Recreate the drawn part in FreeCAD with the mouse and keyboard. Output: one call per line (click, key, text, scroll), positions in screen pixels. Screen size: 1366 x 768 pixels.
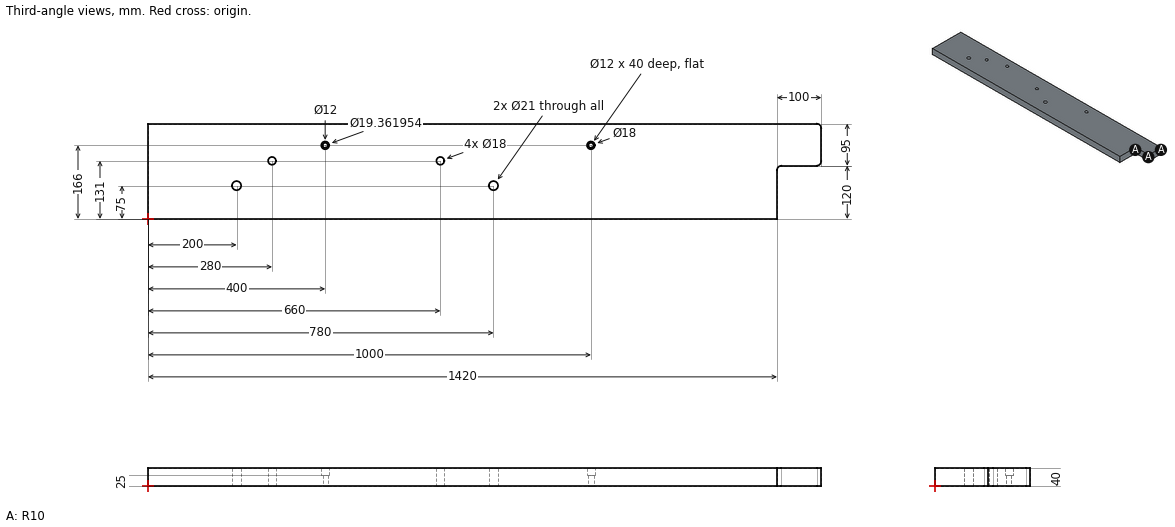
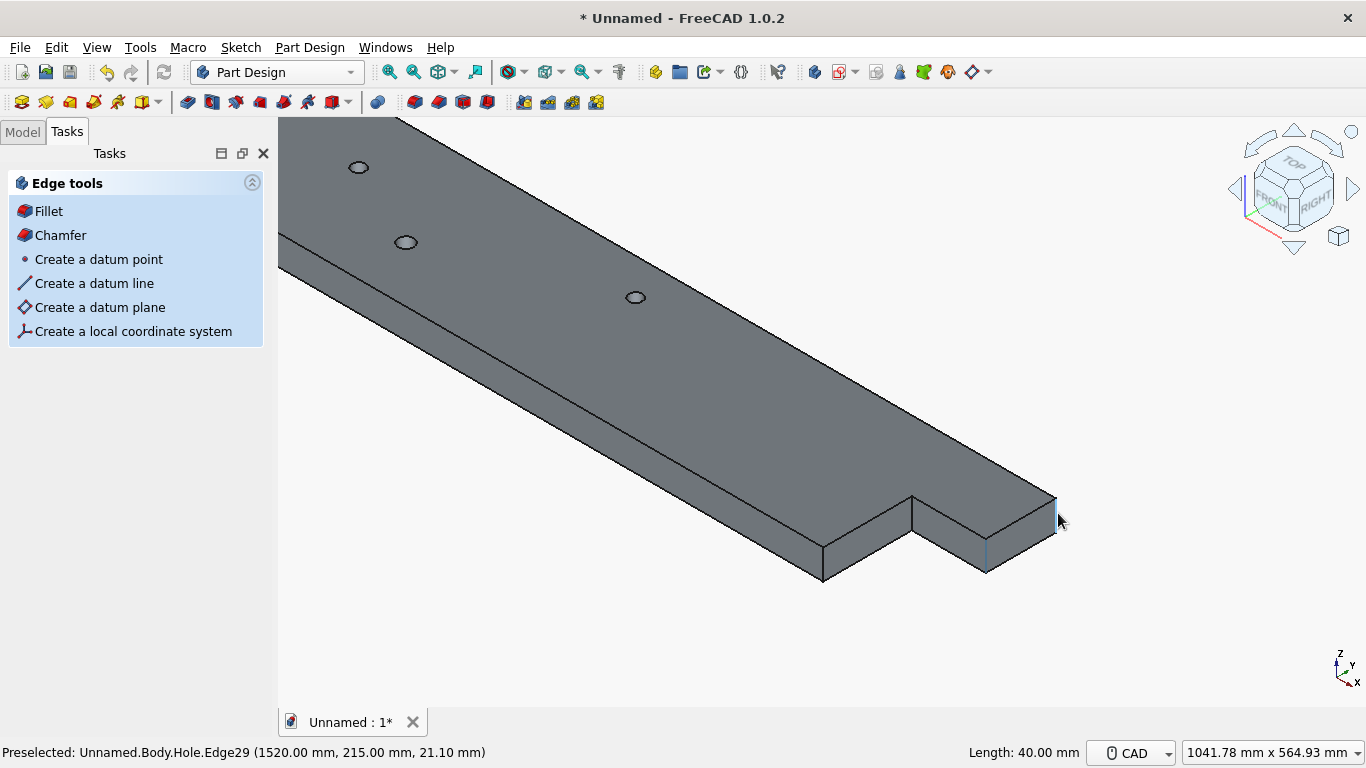
key(v)
key(f)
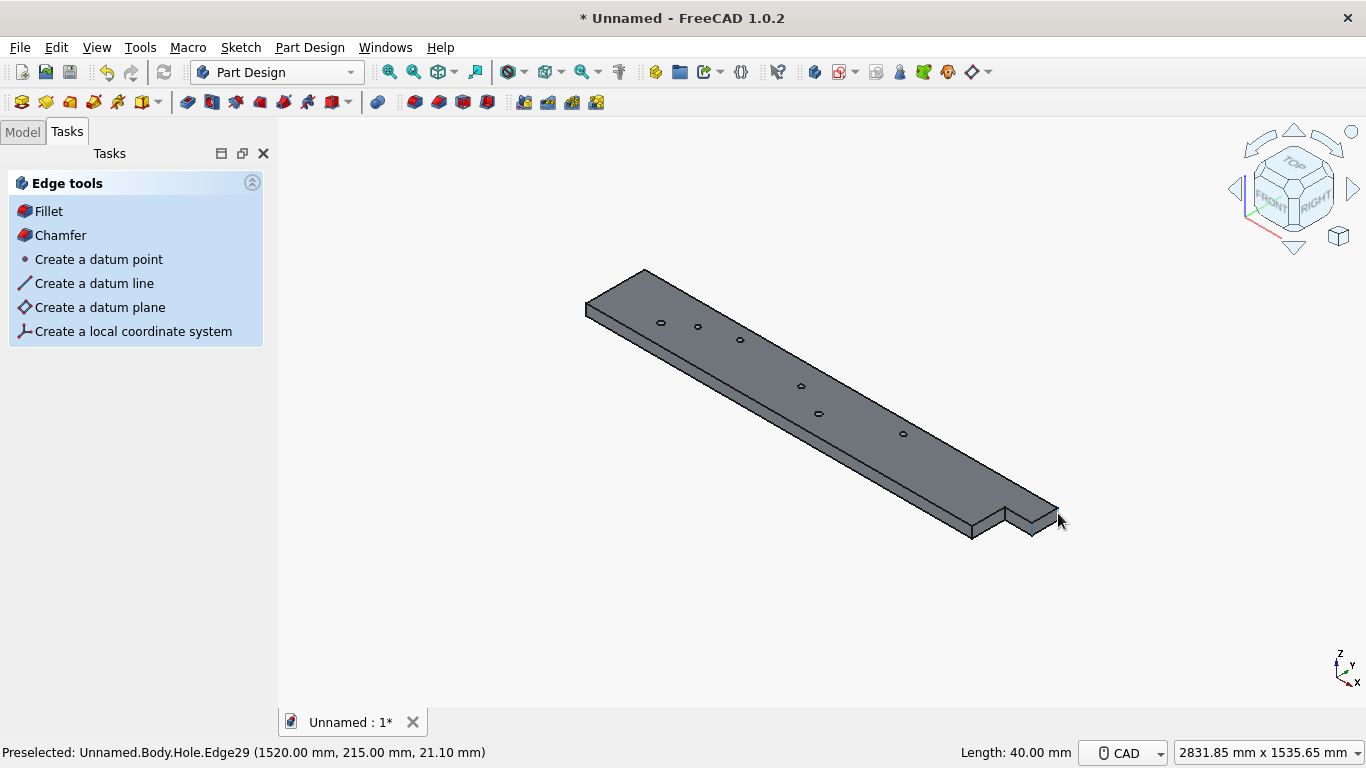
key(2)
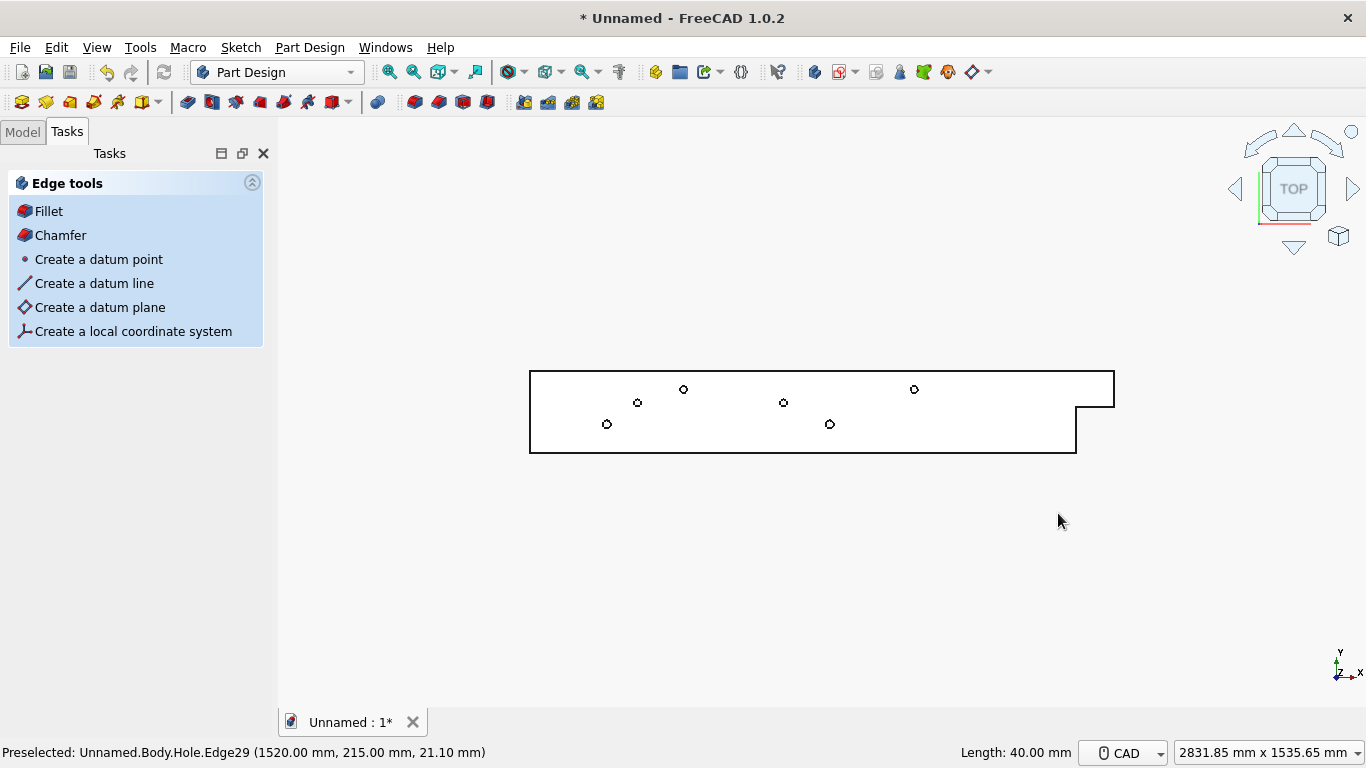
scroll(1114, 370, up, 5)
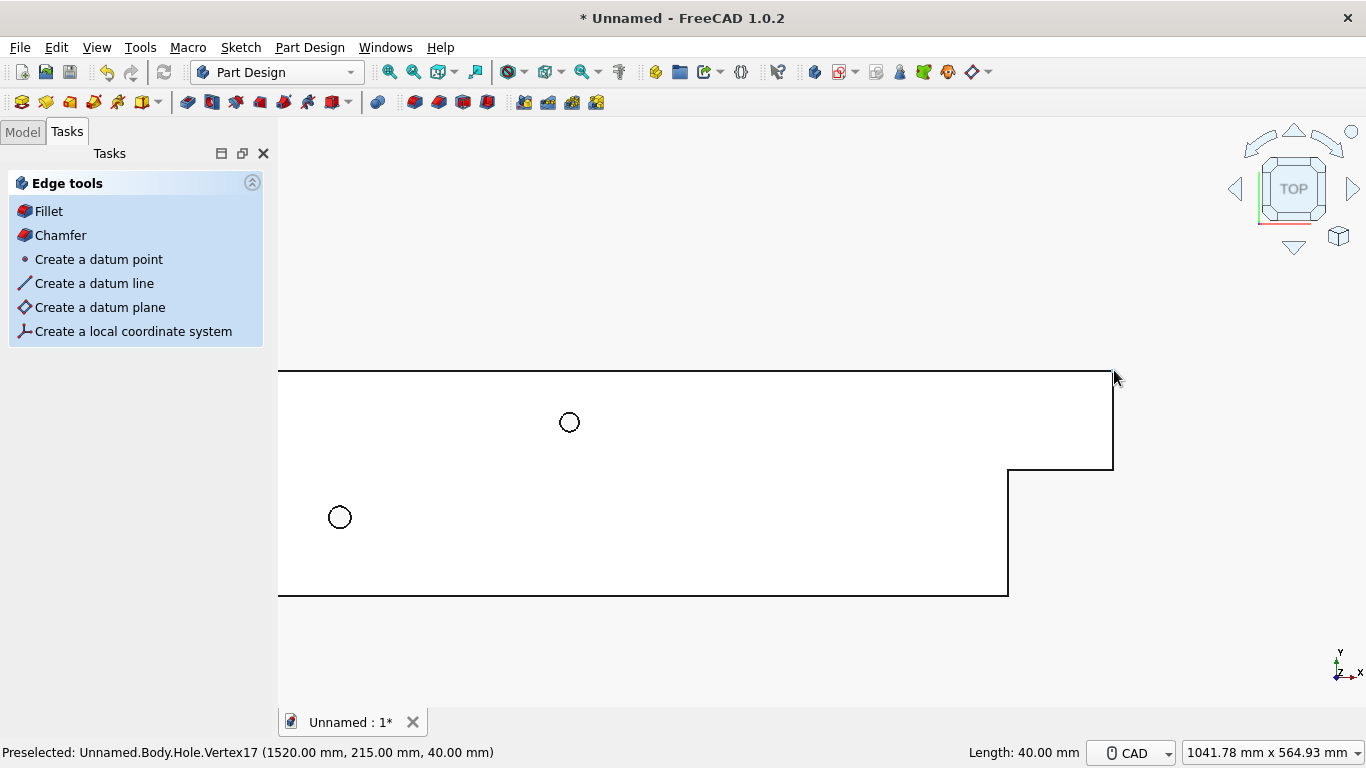
key(v)
key(f)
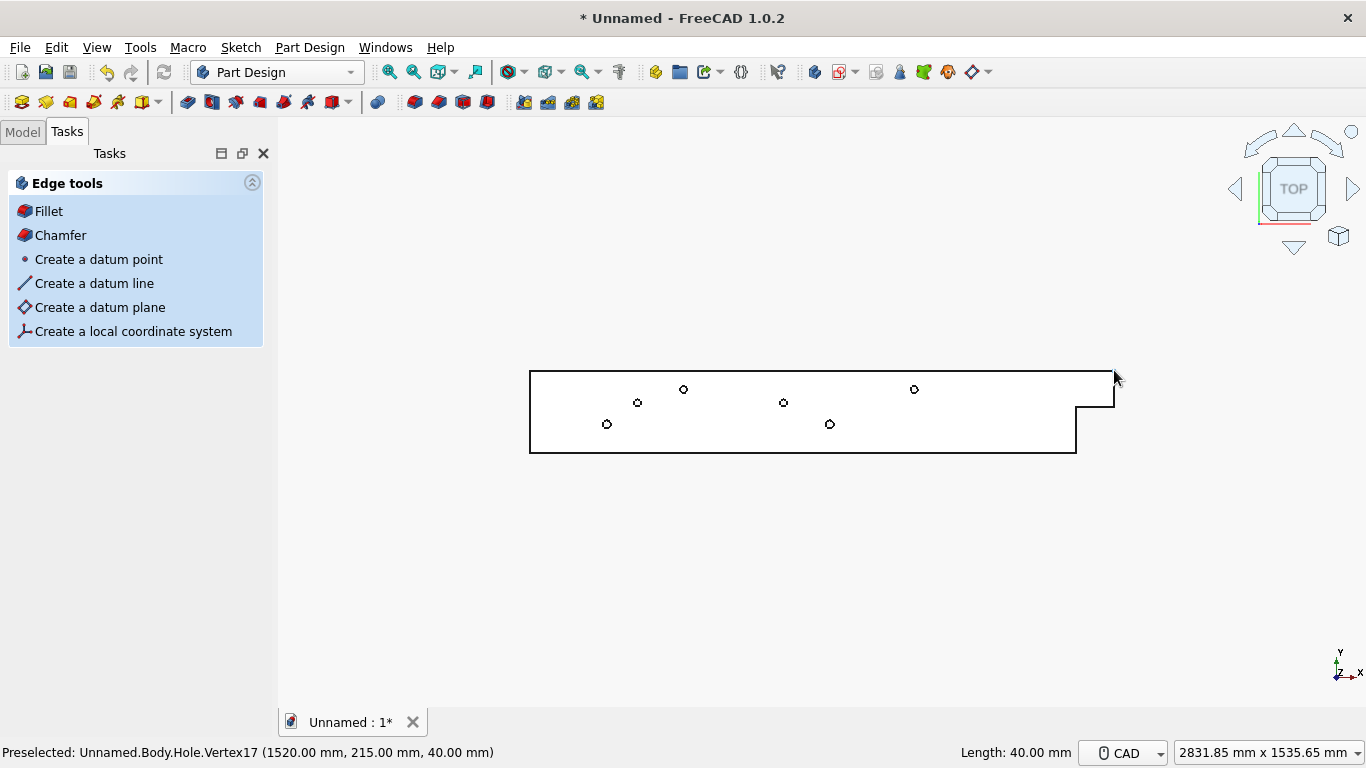
key(1)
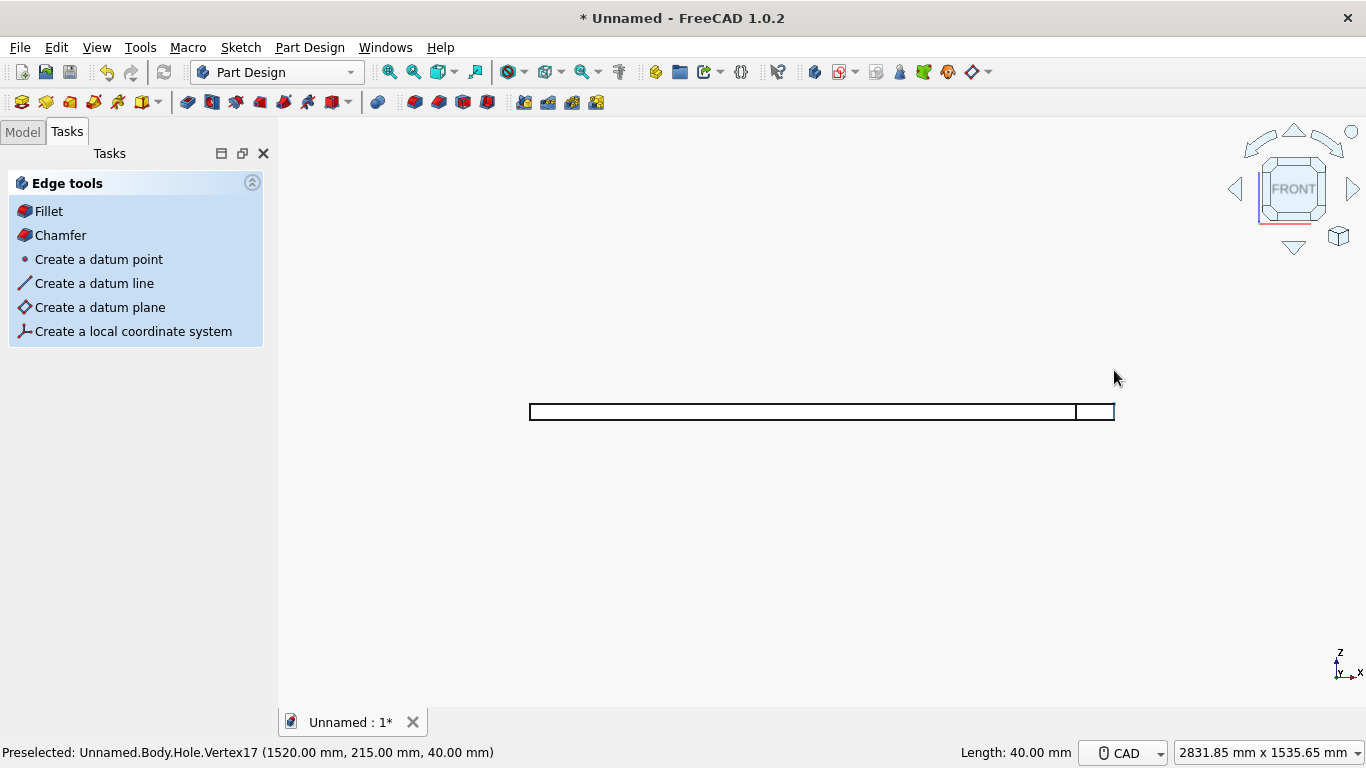
scroll(1114, 411, up, 5)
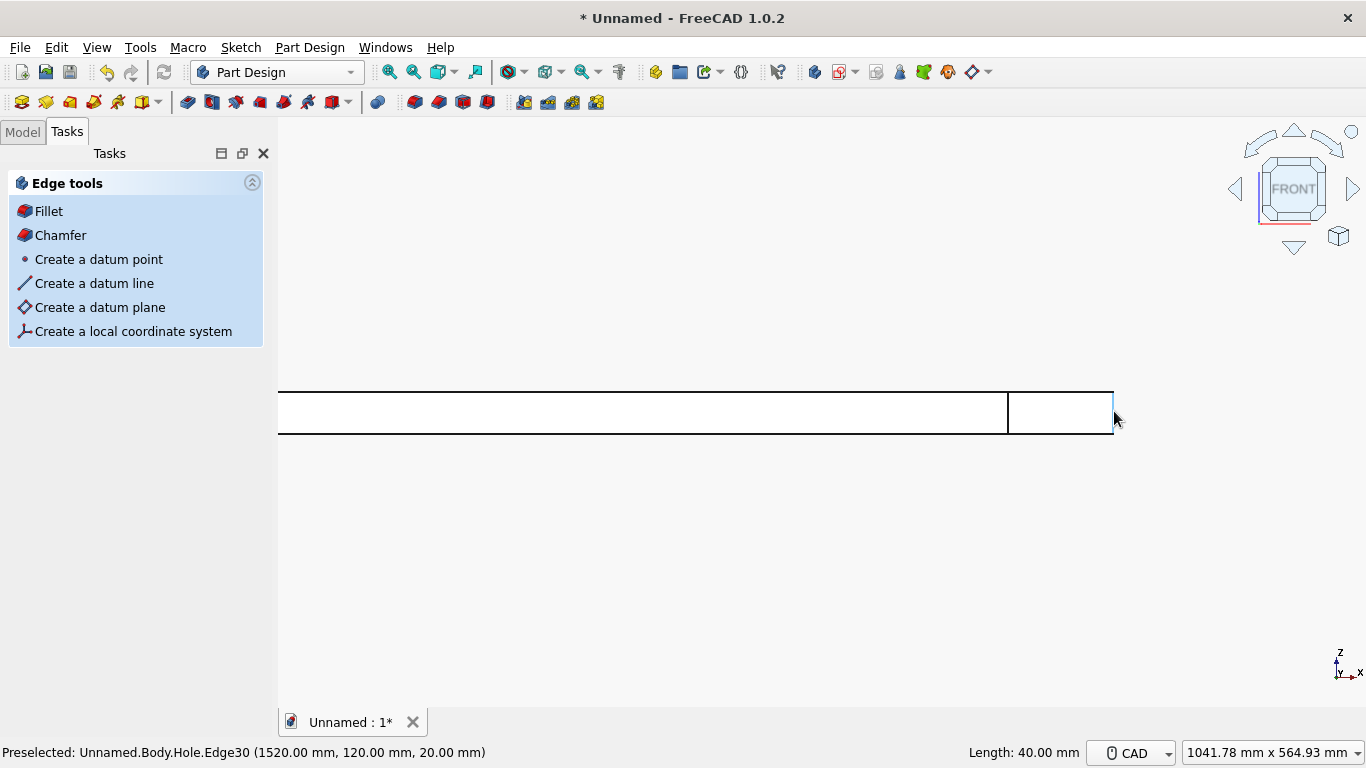
key(v)
key(f)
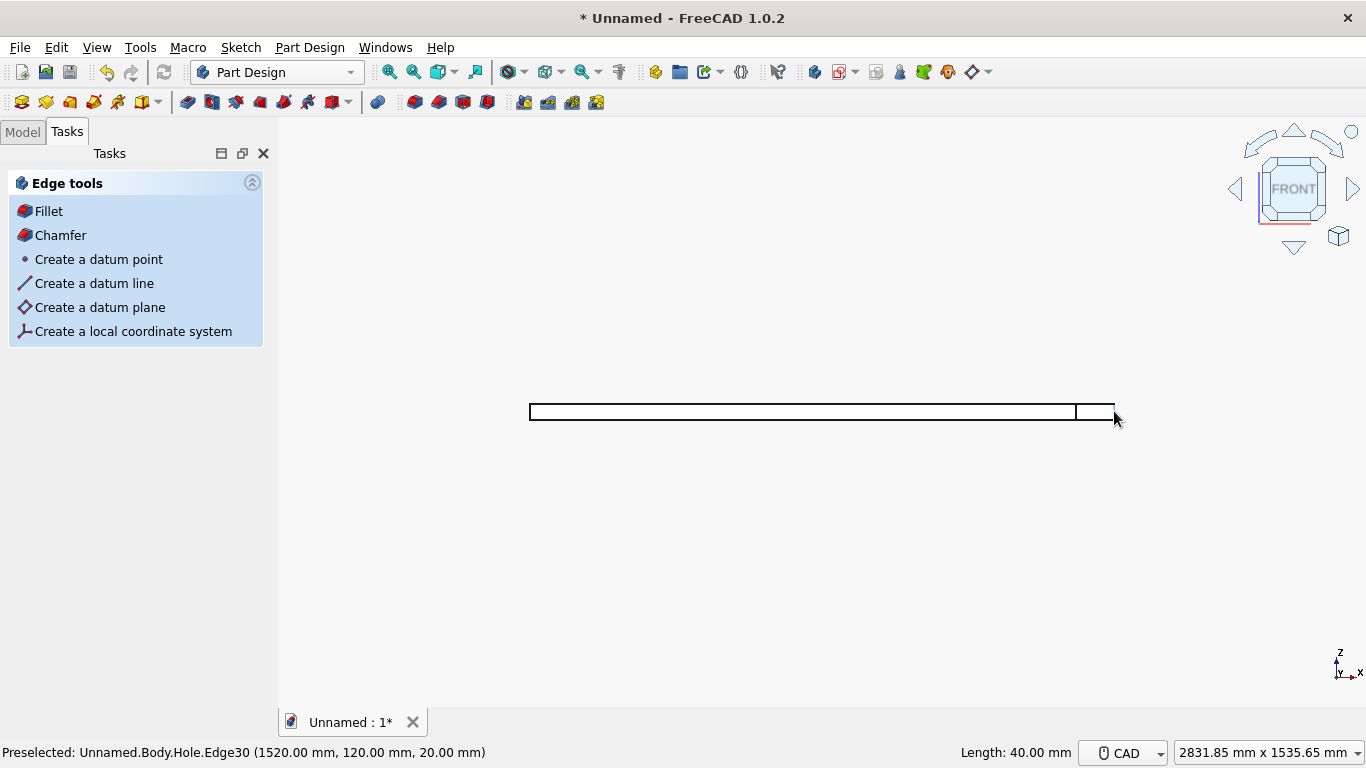
key(3)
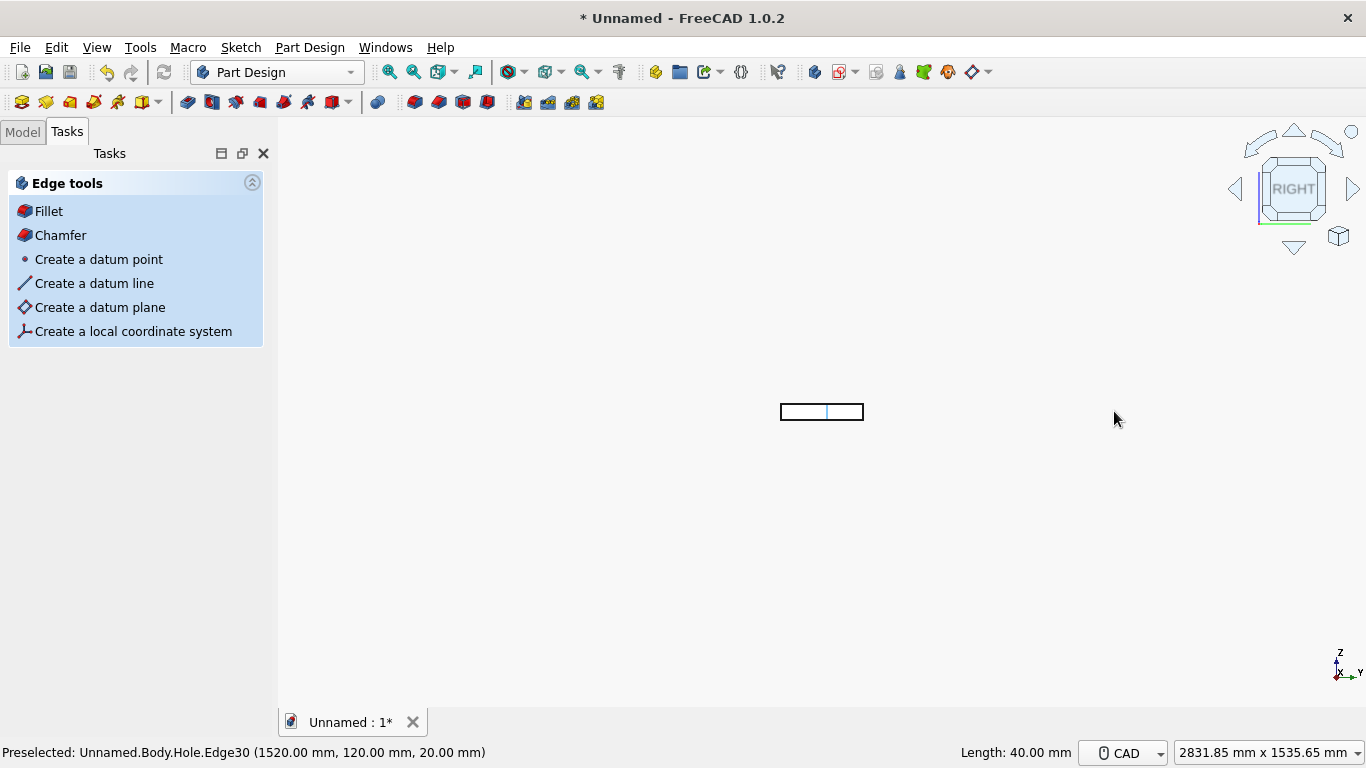
click(390, 72)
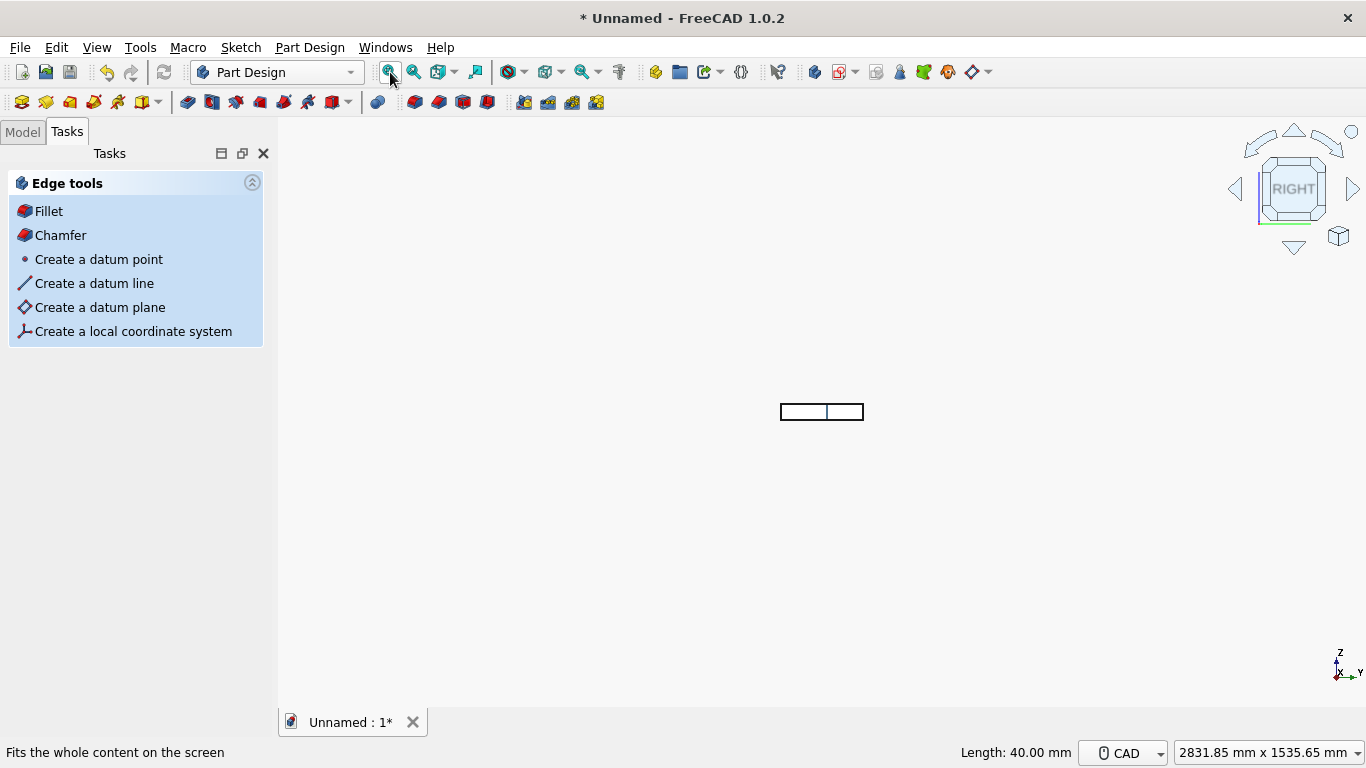
click(863, 411, ctrl)